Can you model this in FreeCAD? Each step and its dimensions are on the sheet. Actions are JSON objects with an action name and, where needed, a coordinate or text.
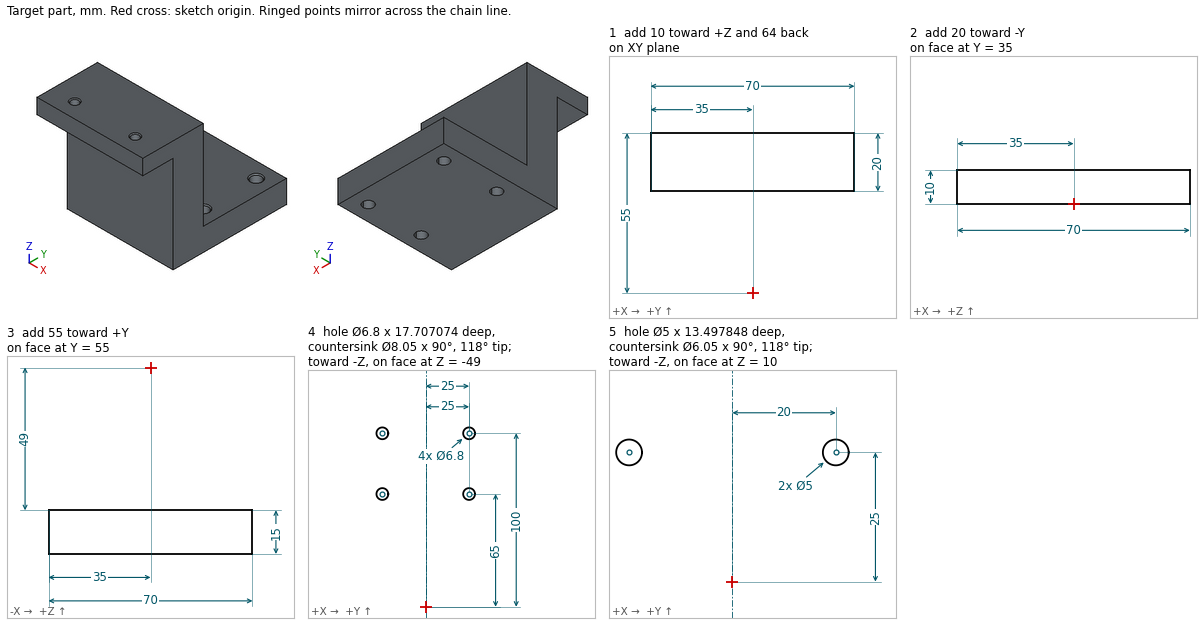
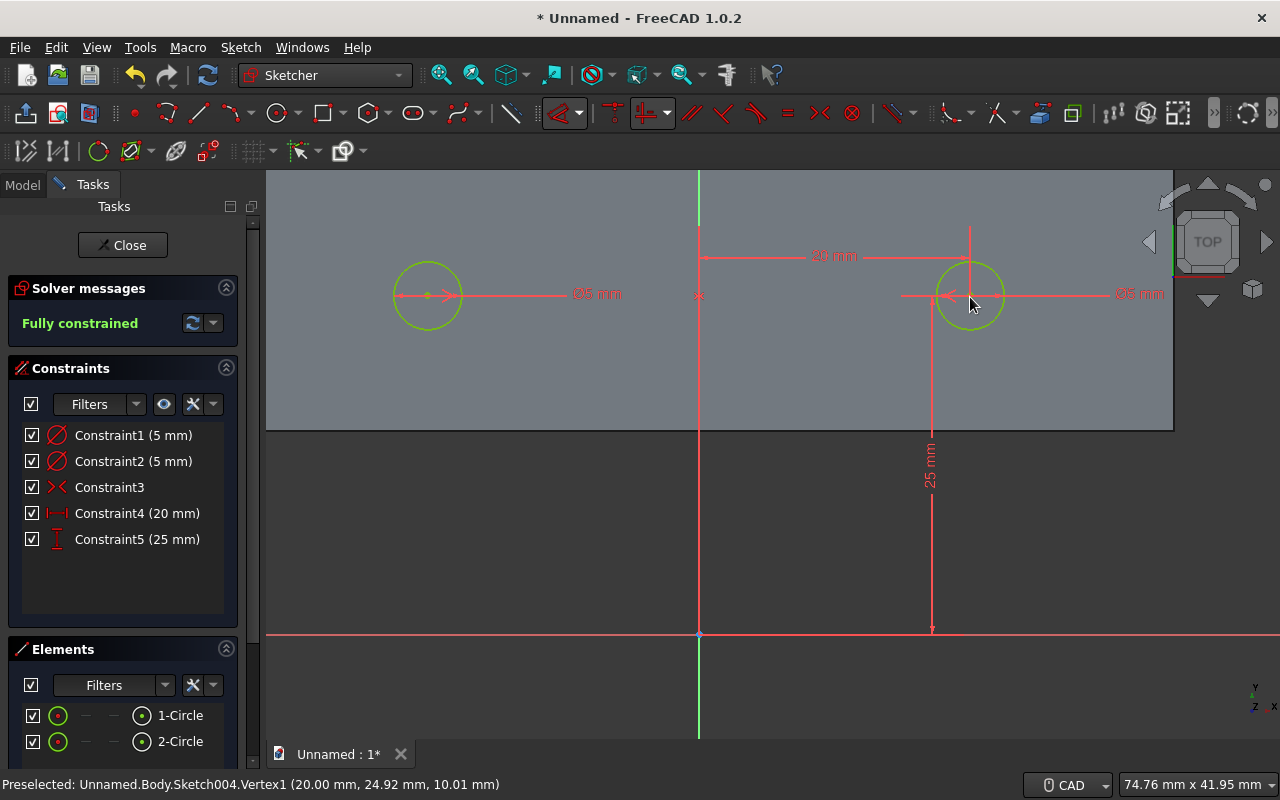
{"action": "left_click", "coordinate": [123, 245]}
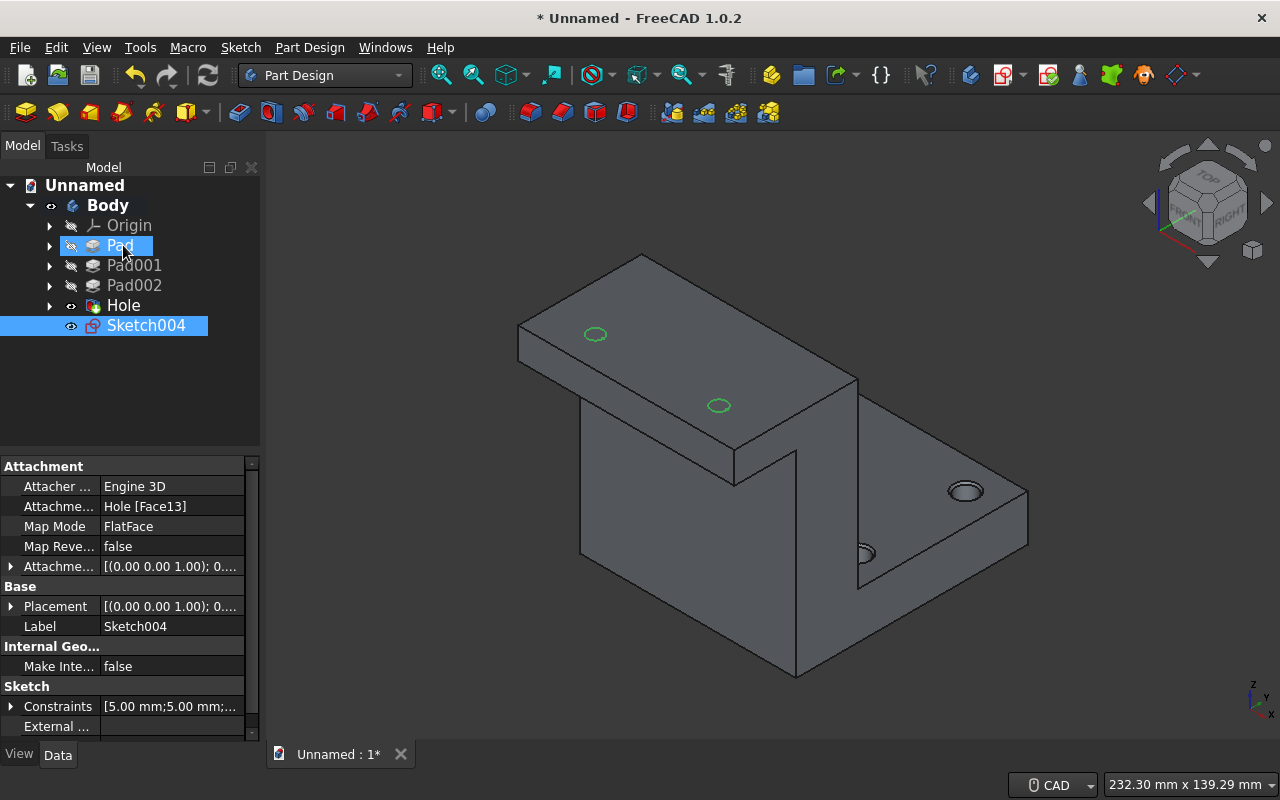
{"action": "left_click", "coordinate": [272, 112]}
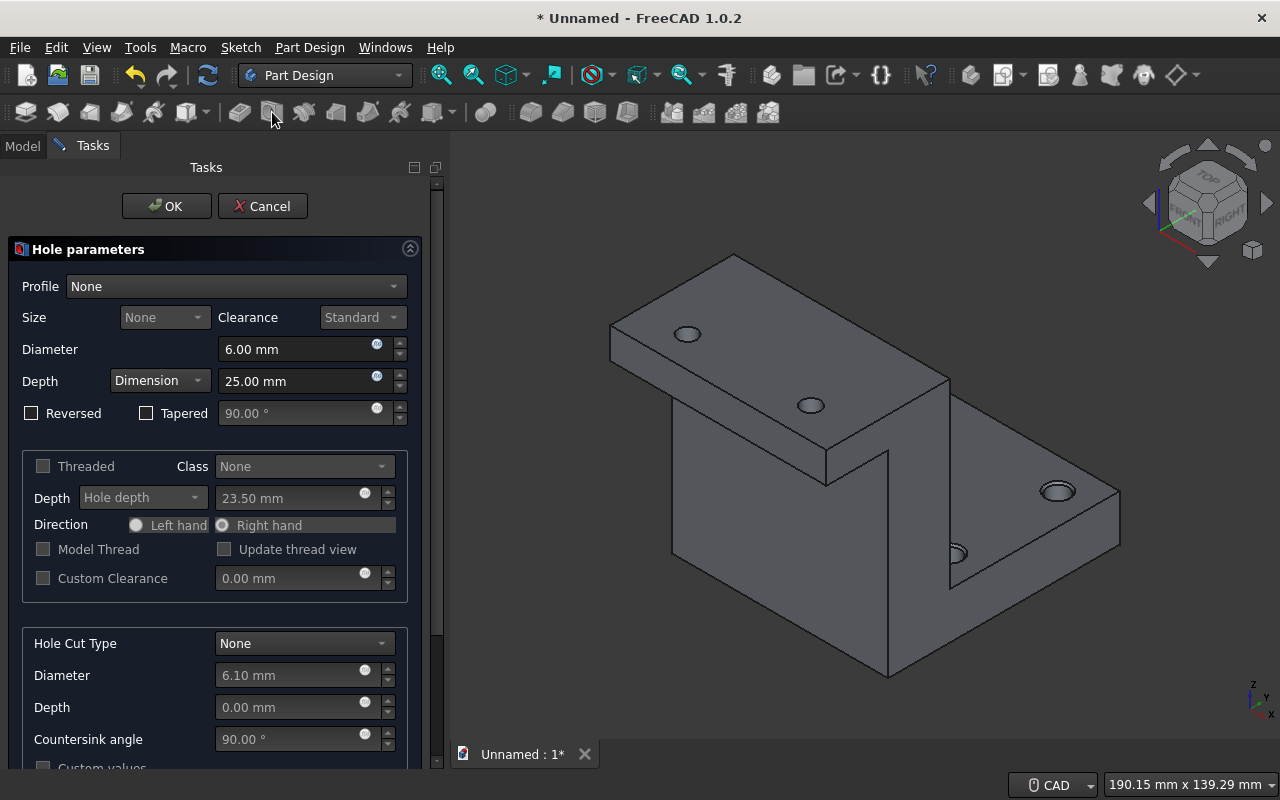
{"action": "triple_click", "coordinate": [305, 349]}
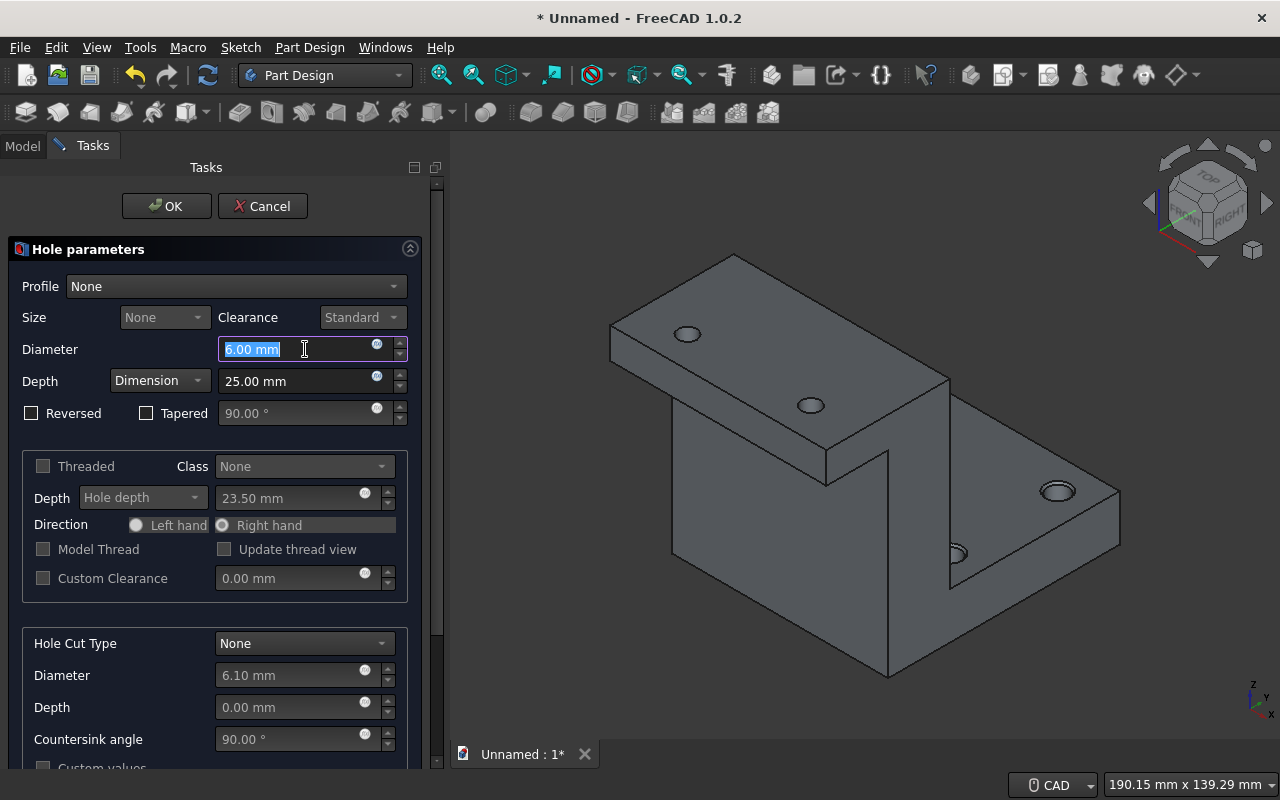
{"action": "type", "text": "5"}
{"action": "key", "text": "Tab"}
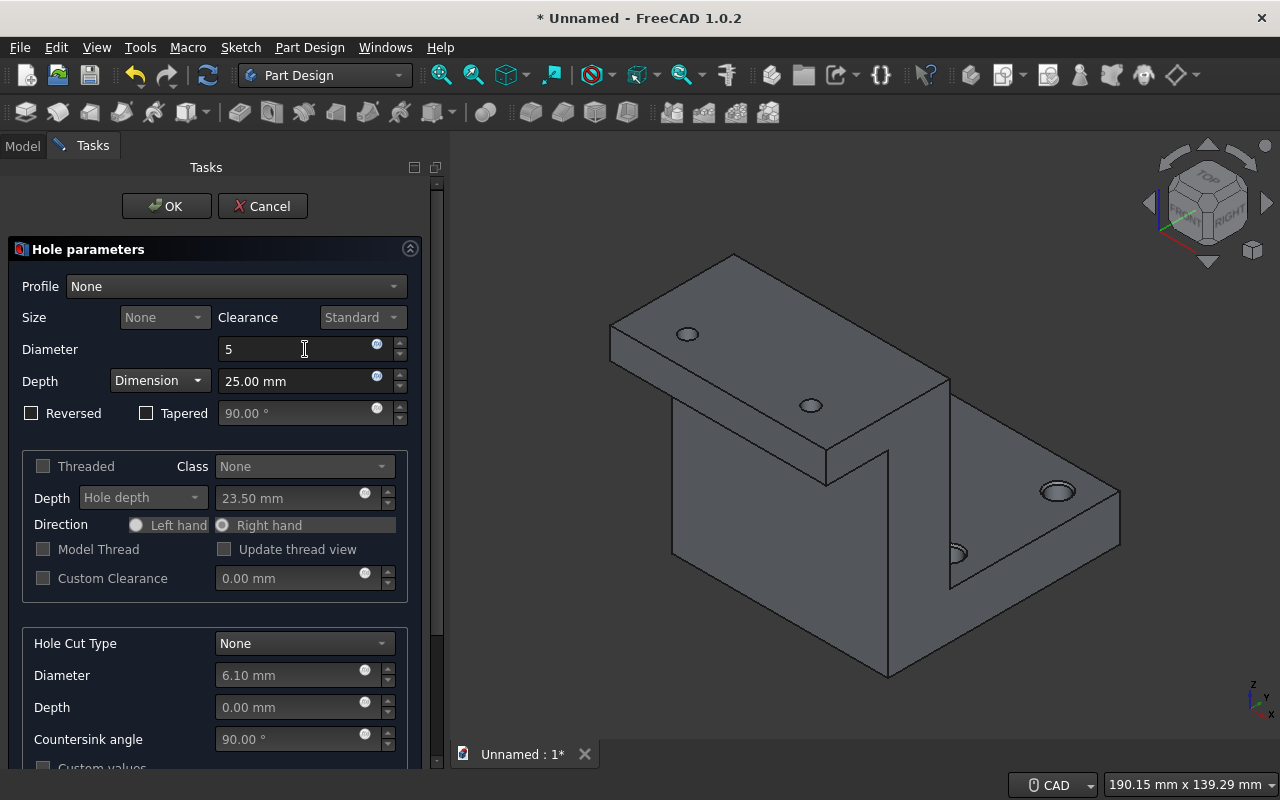
{"action": "triple_click", "coordinate": [305, 381]}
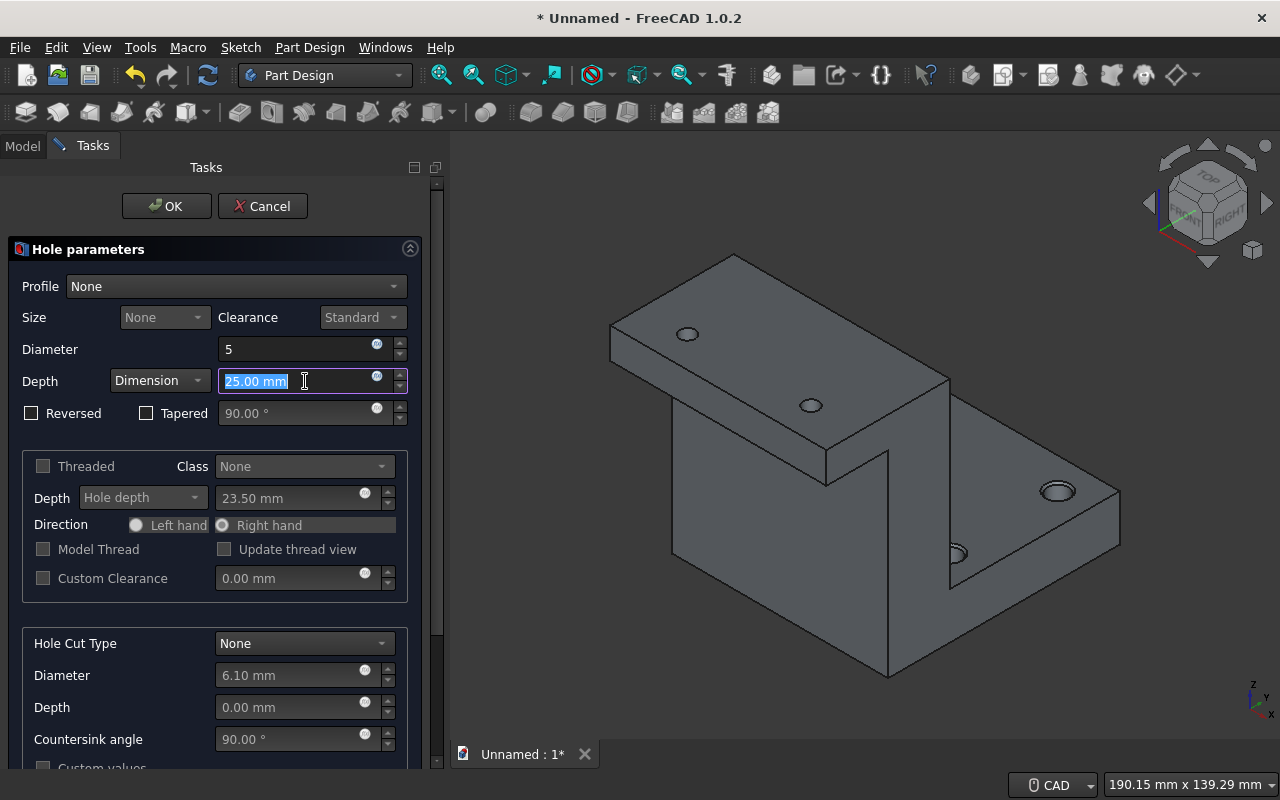
{"action": "type", "text": "13.497848"}
{"action": "key", "text": "Tab"}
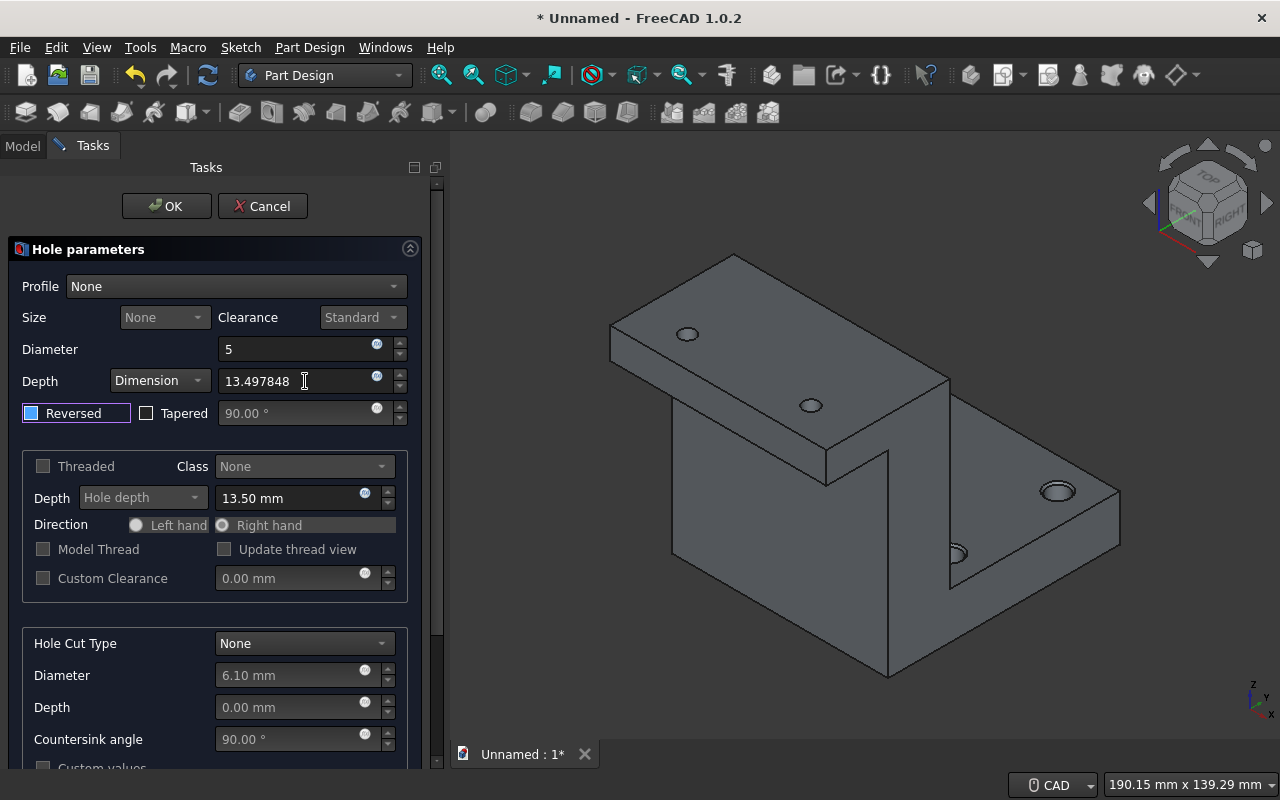
{"action": "left_click", "coordinate": [306, 644]}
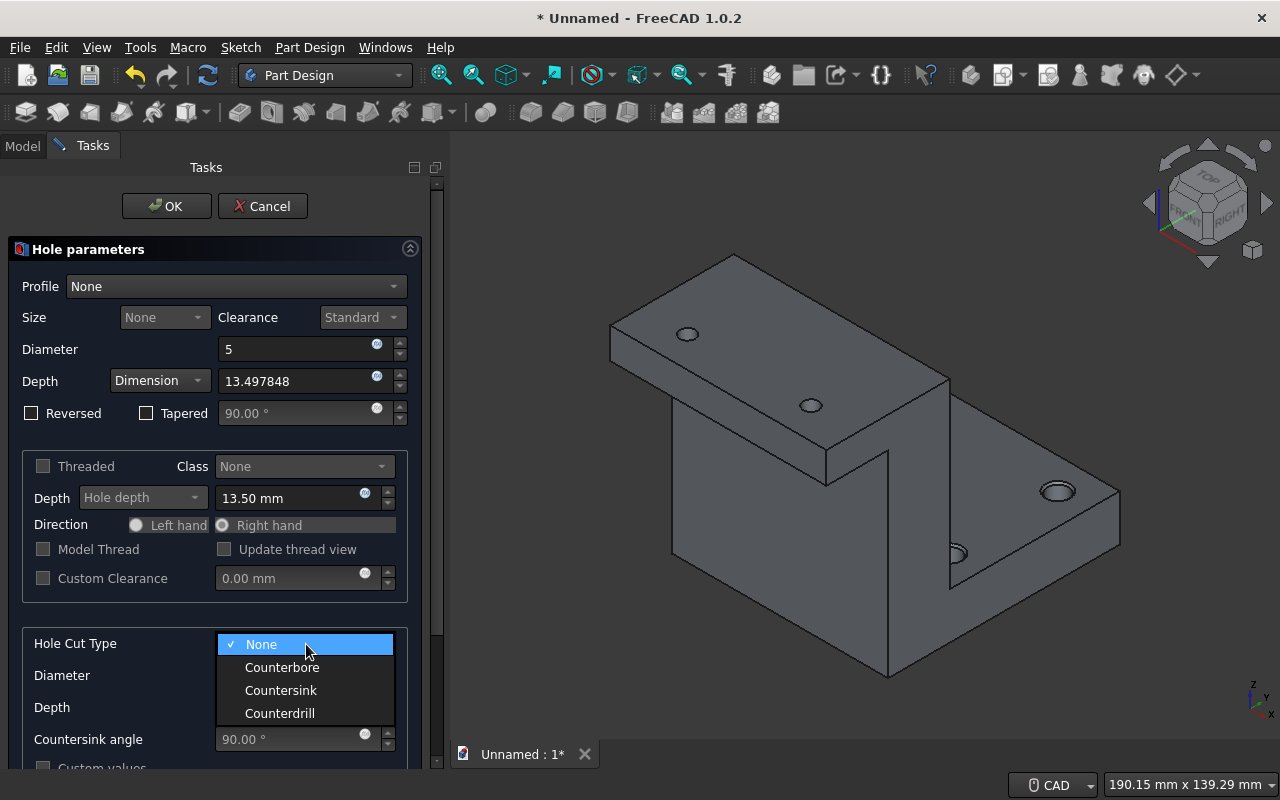
{"action": "left_click", "coordinate": [304, 690]}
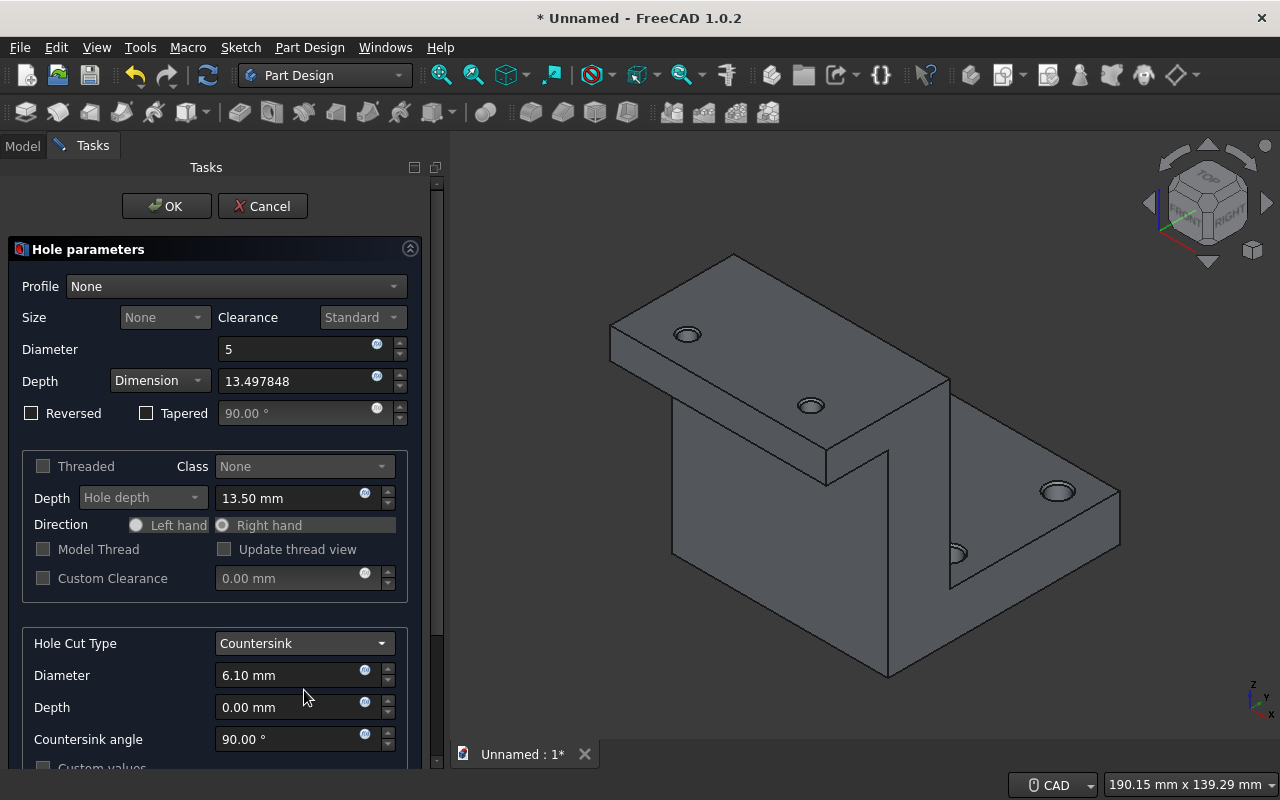
{"action": "triple_click", "coordinate": [298, 675]}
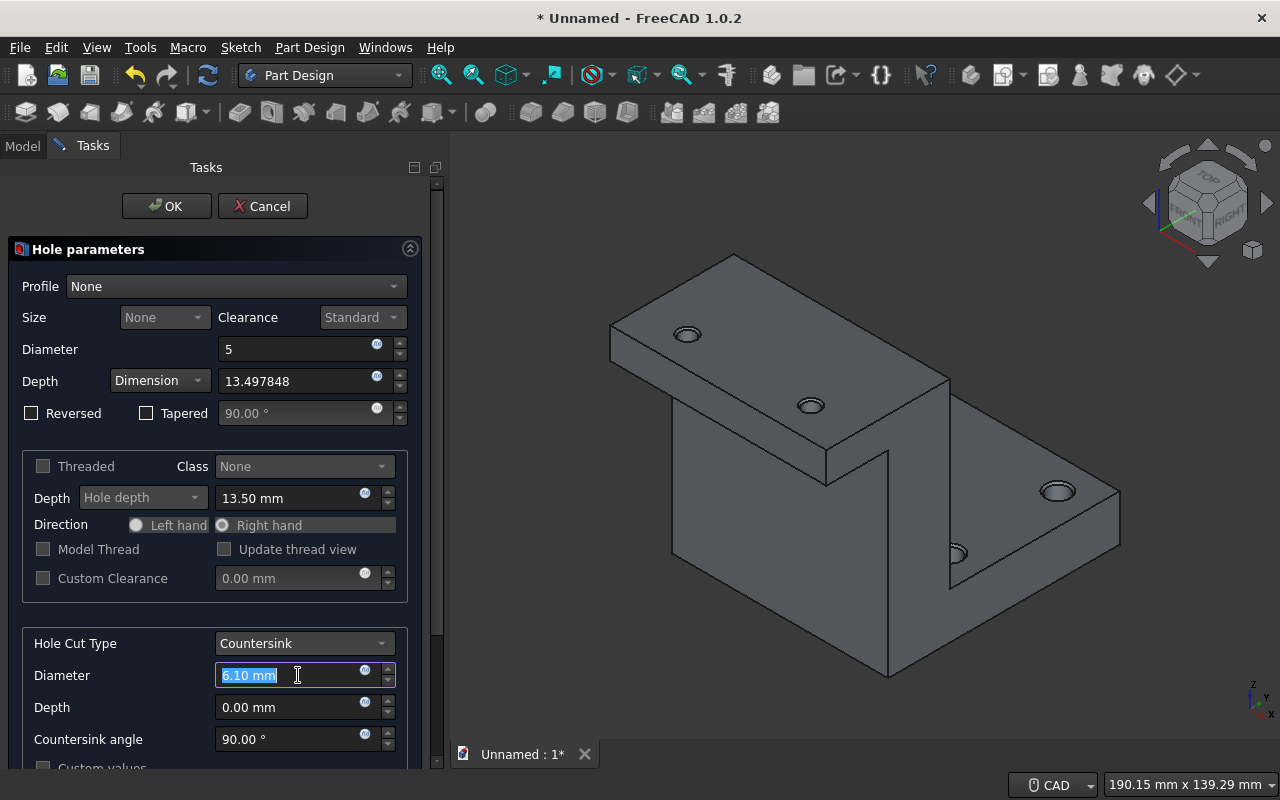
{"action": "type", "text": "6.05"}
{"action": "key", "text": "Tab"}